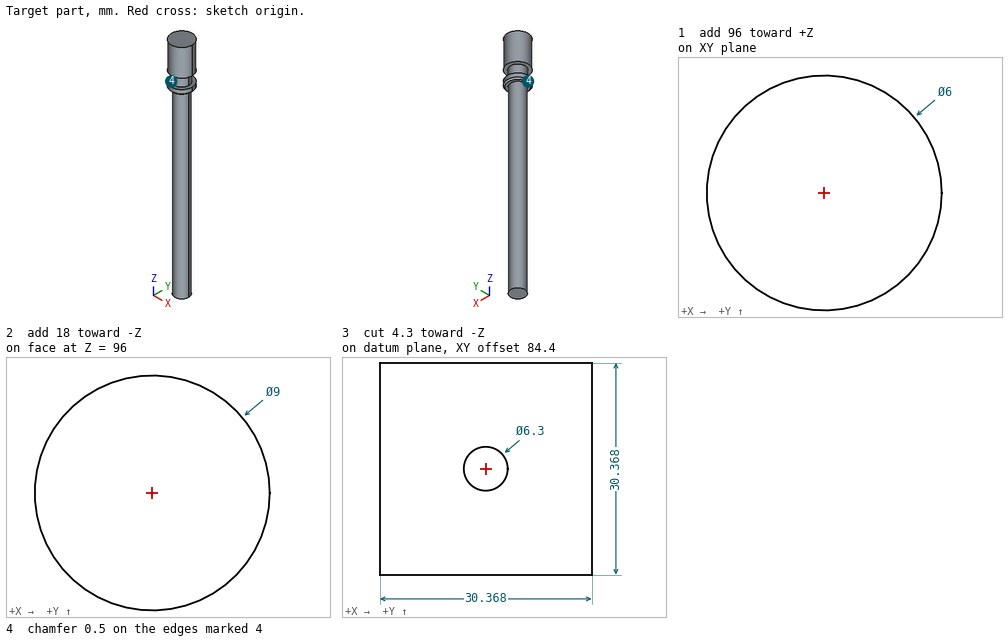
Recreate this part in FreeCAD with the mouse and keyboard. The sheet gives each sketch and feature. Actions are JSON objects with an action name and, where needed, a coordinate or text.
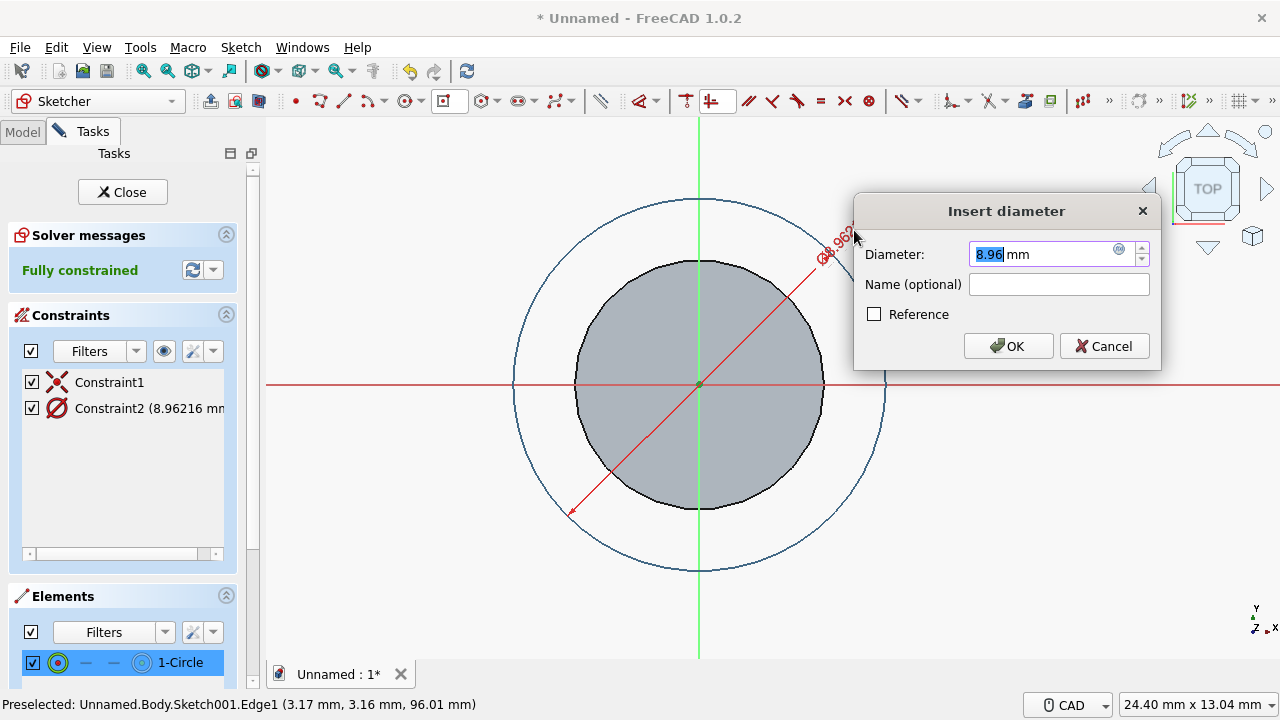
{"action": "type", "text": "9"}
{"action": "key", "text": "Return"}
{"action": "key", "text": "Escape"}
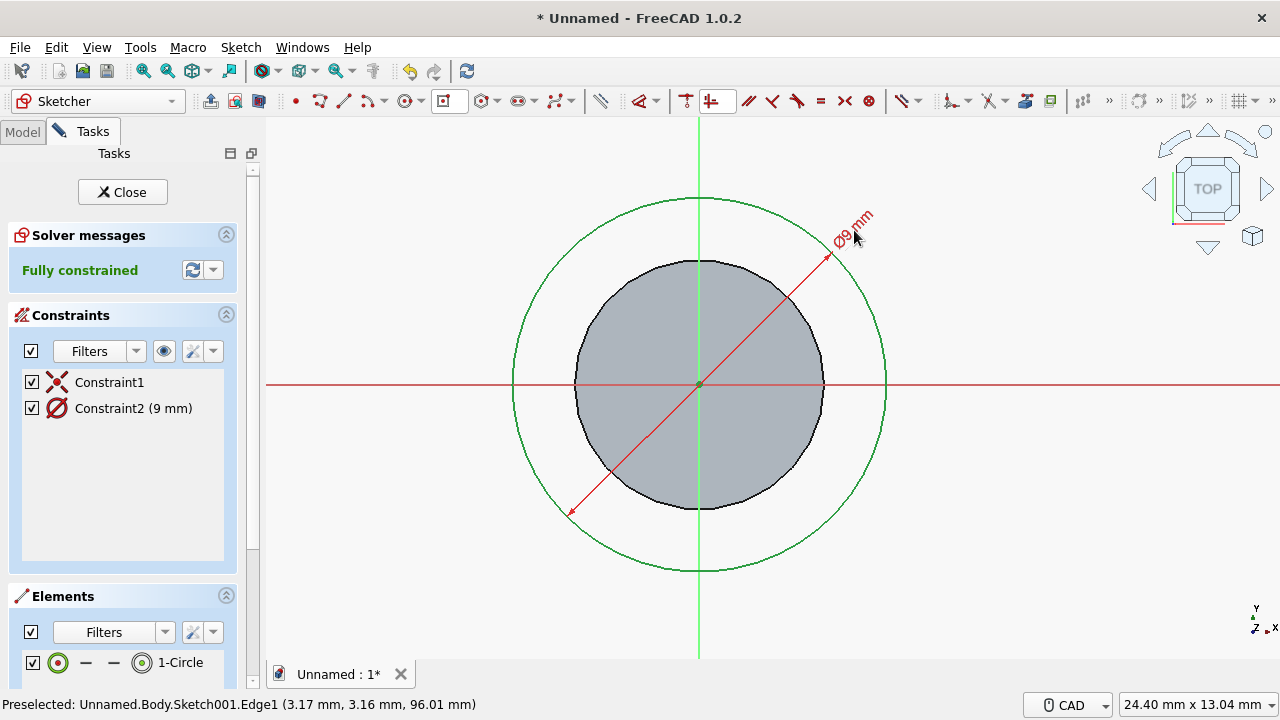
{"action": "left_click", "coordinate": [123, 192]}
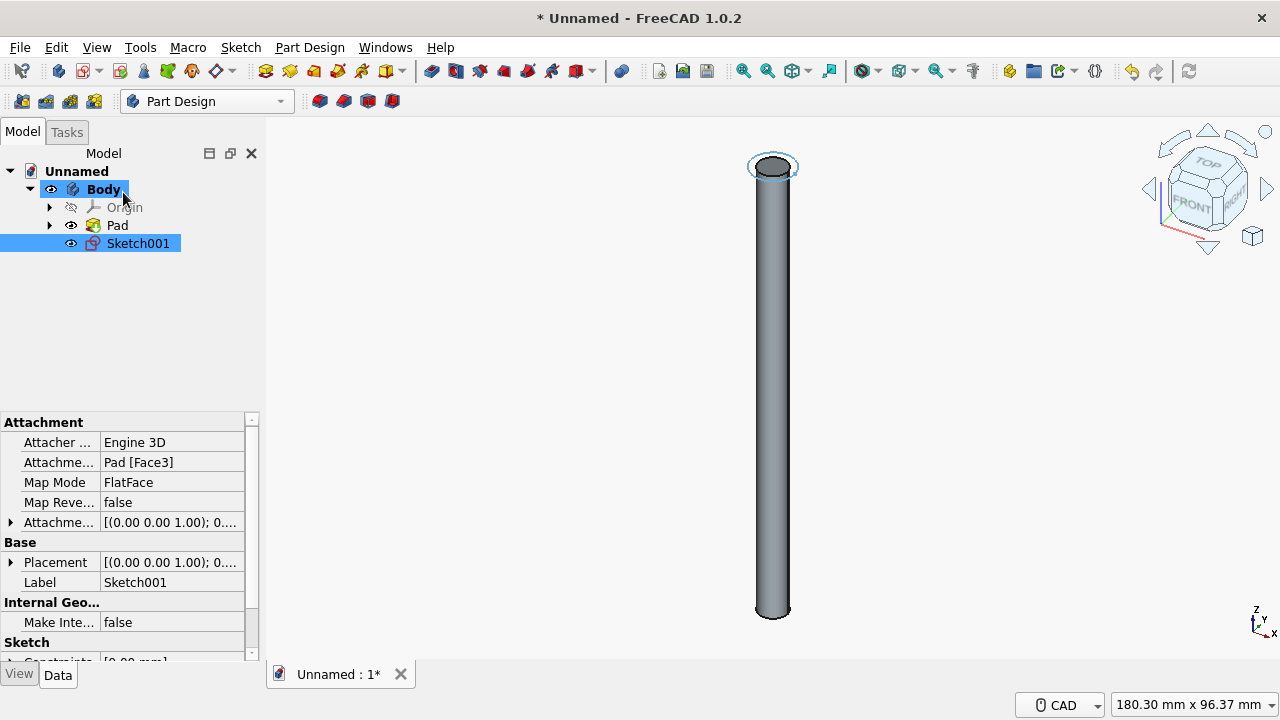
{"action": "left_click", "coordinate": [266, 72]}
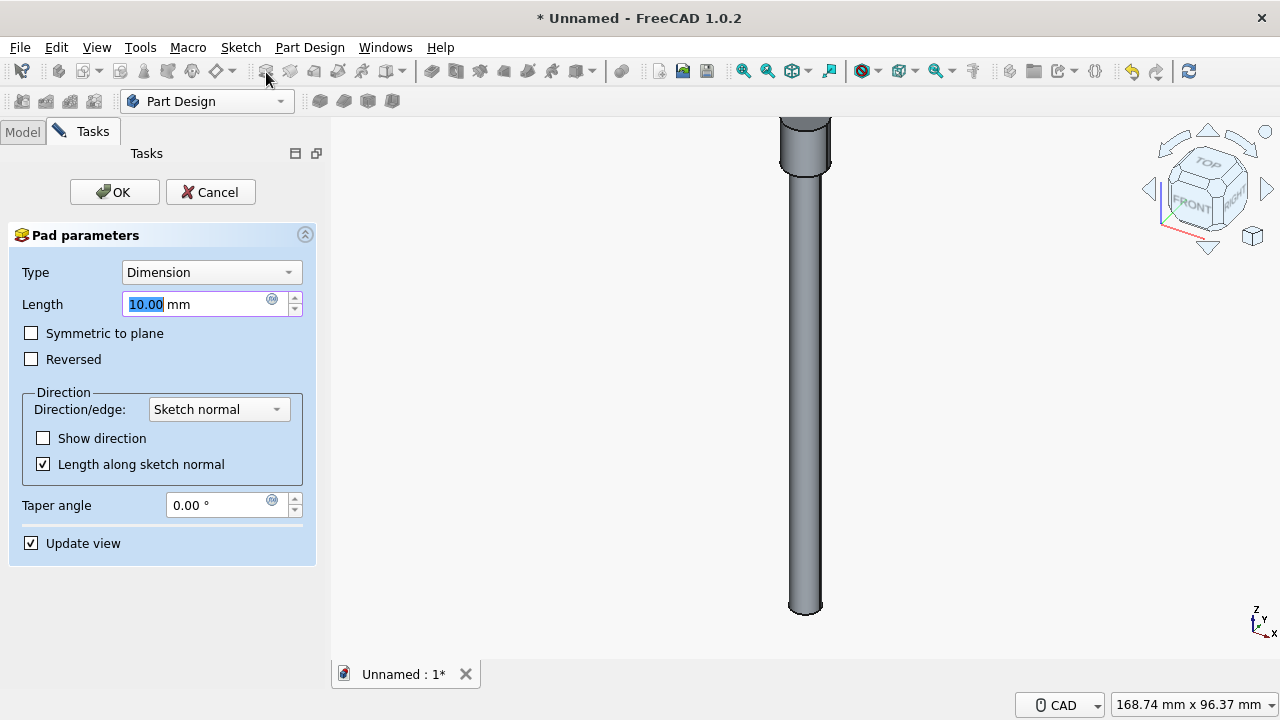
{"action": "type", "text": "18"}
{"action": "key", "text": "Tab"}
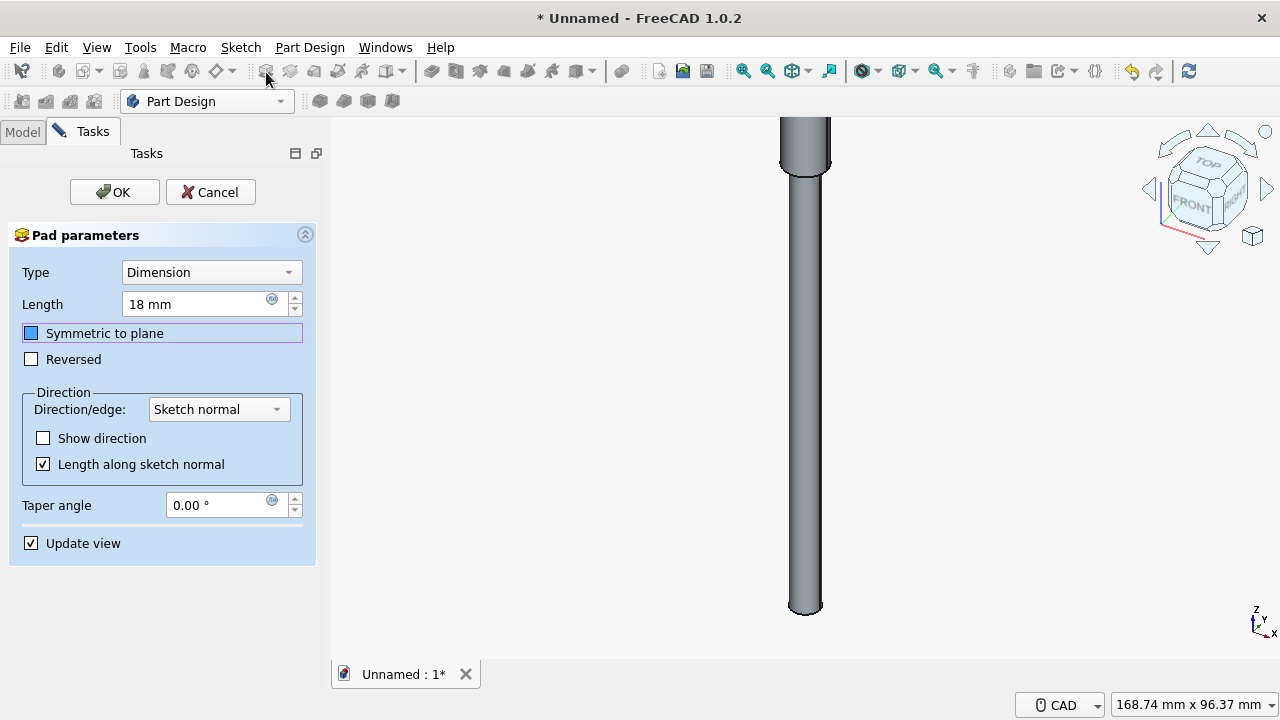
{"action": "left_click", "coordinate": [30, 359]}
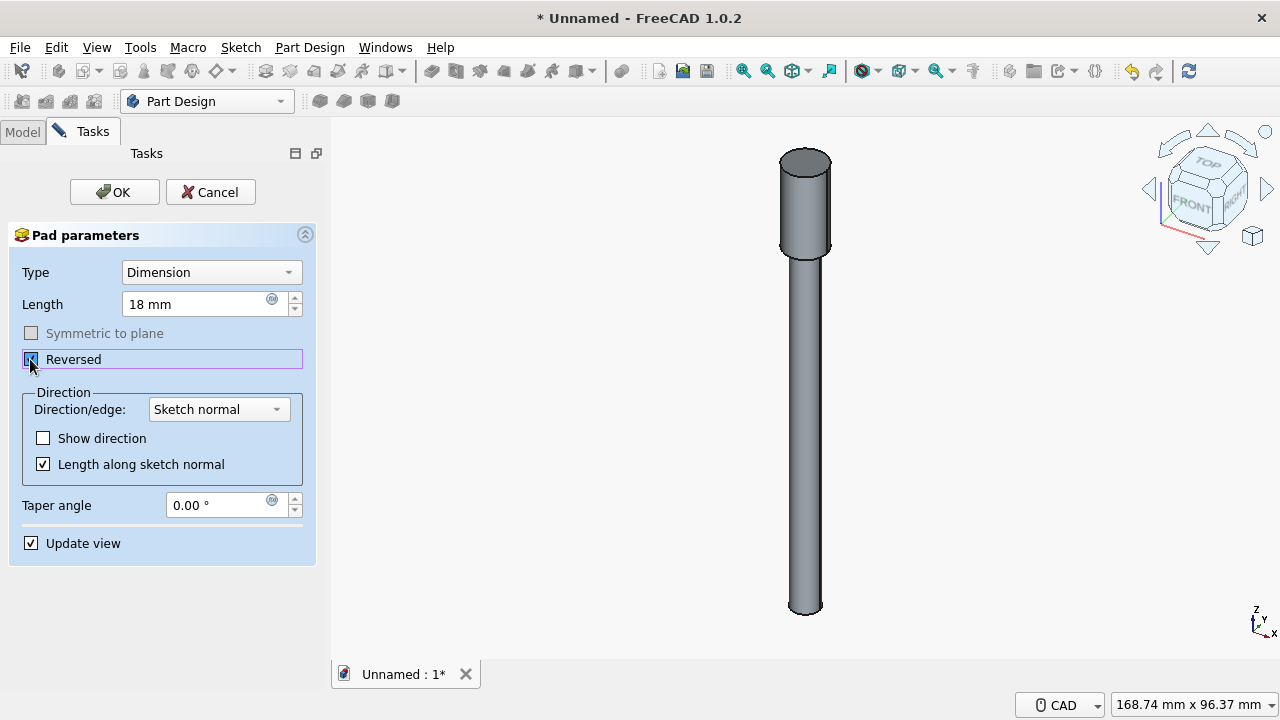
{"action": "left_click", "coordinate": [115, 192]}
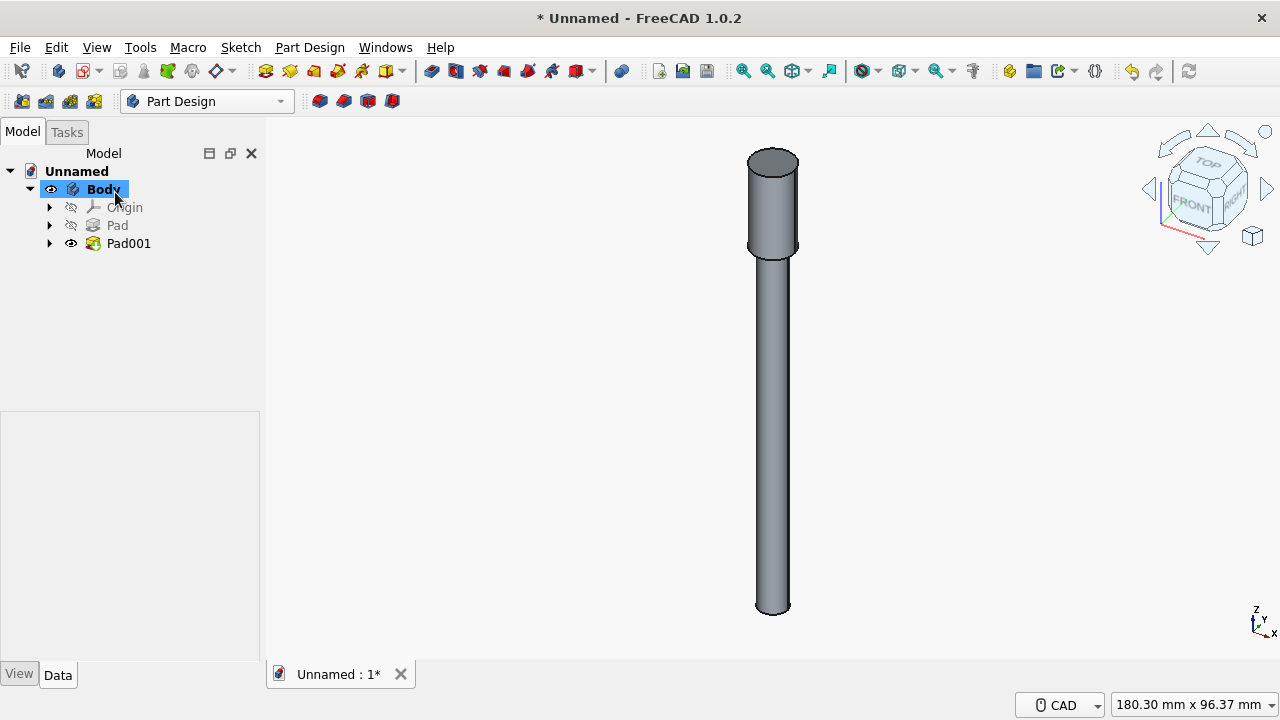
{"action": "left_click", "coordinate": [50, 207]}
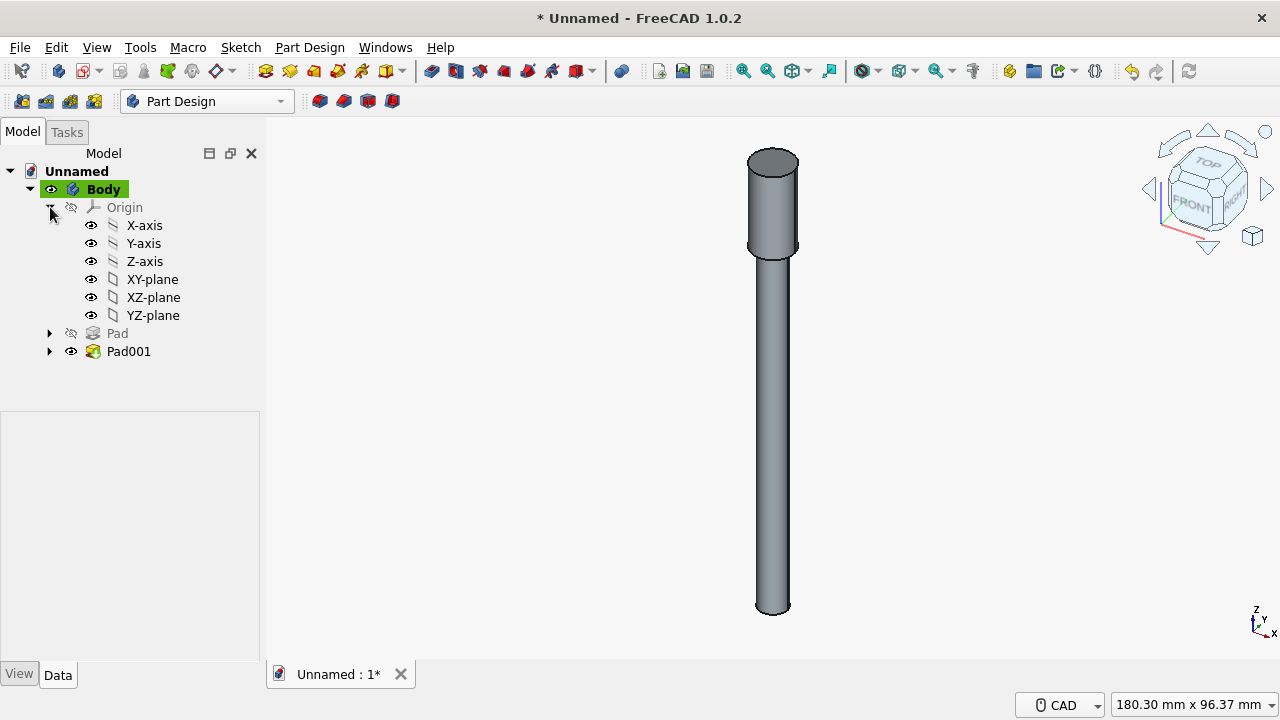
{"action": "left_click", "coordinate": [136, 279]}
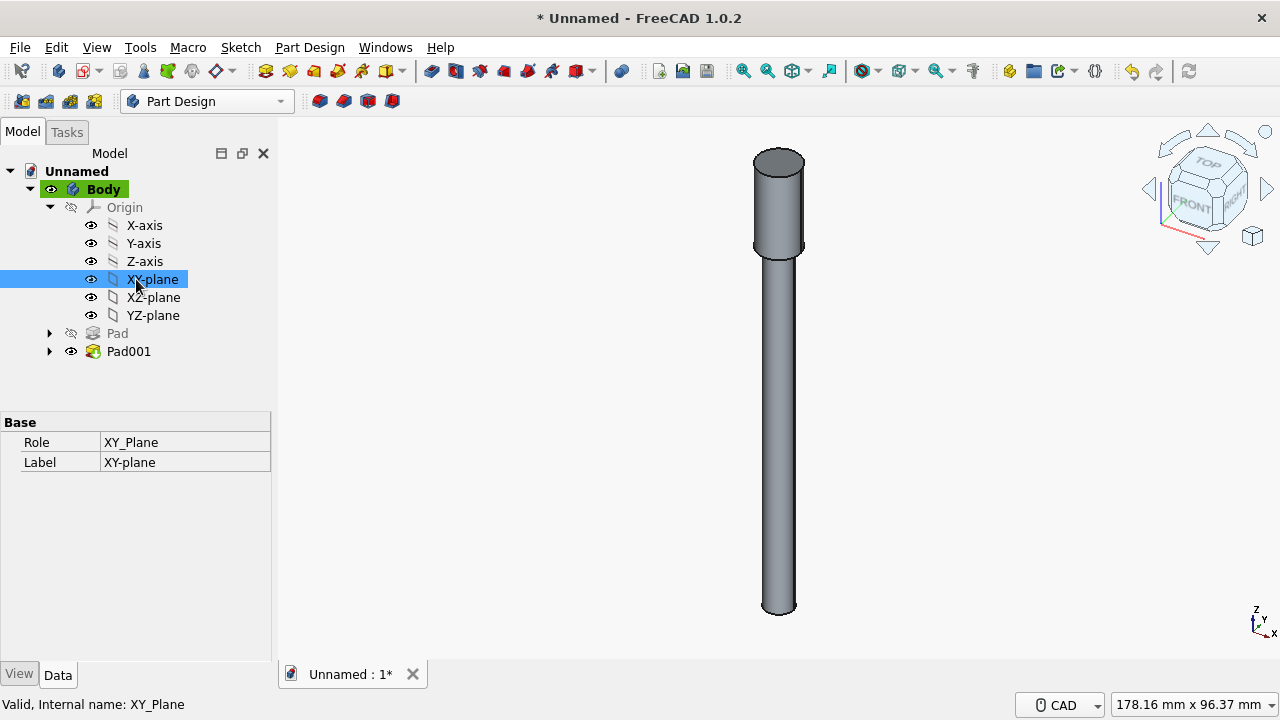
{"action": "left_click", "coordinate": [216, 72]}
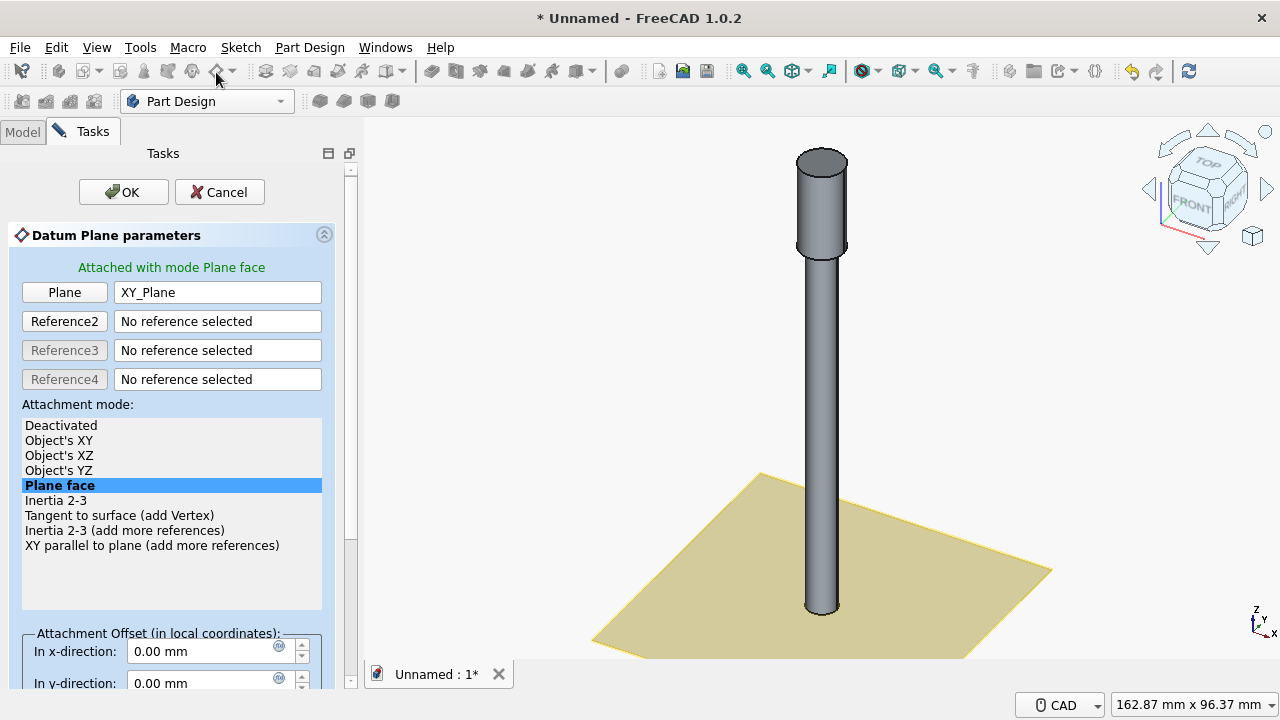
{"action": "scroll", "coordinate": [351, 426], "scroll_direction": "down", "scroll_amount": 2}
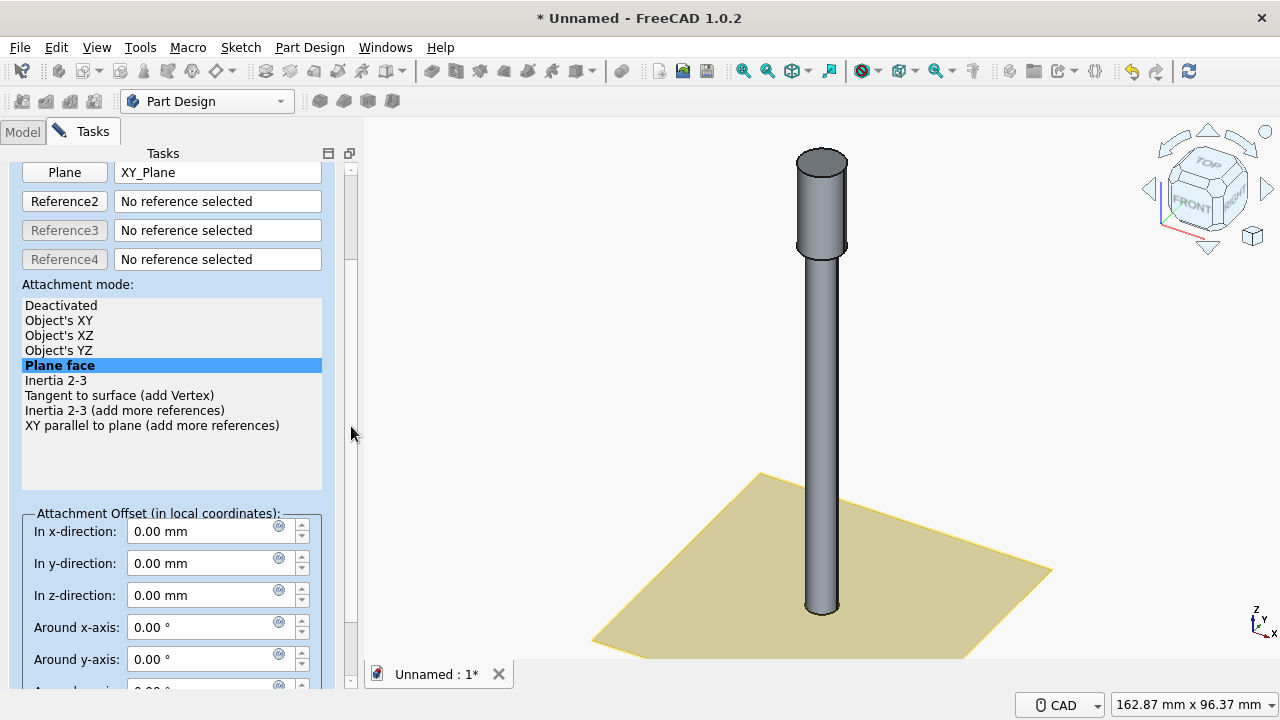
{"action": "triple_click", "coordinate": [210, 595]}